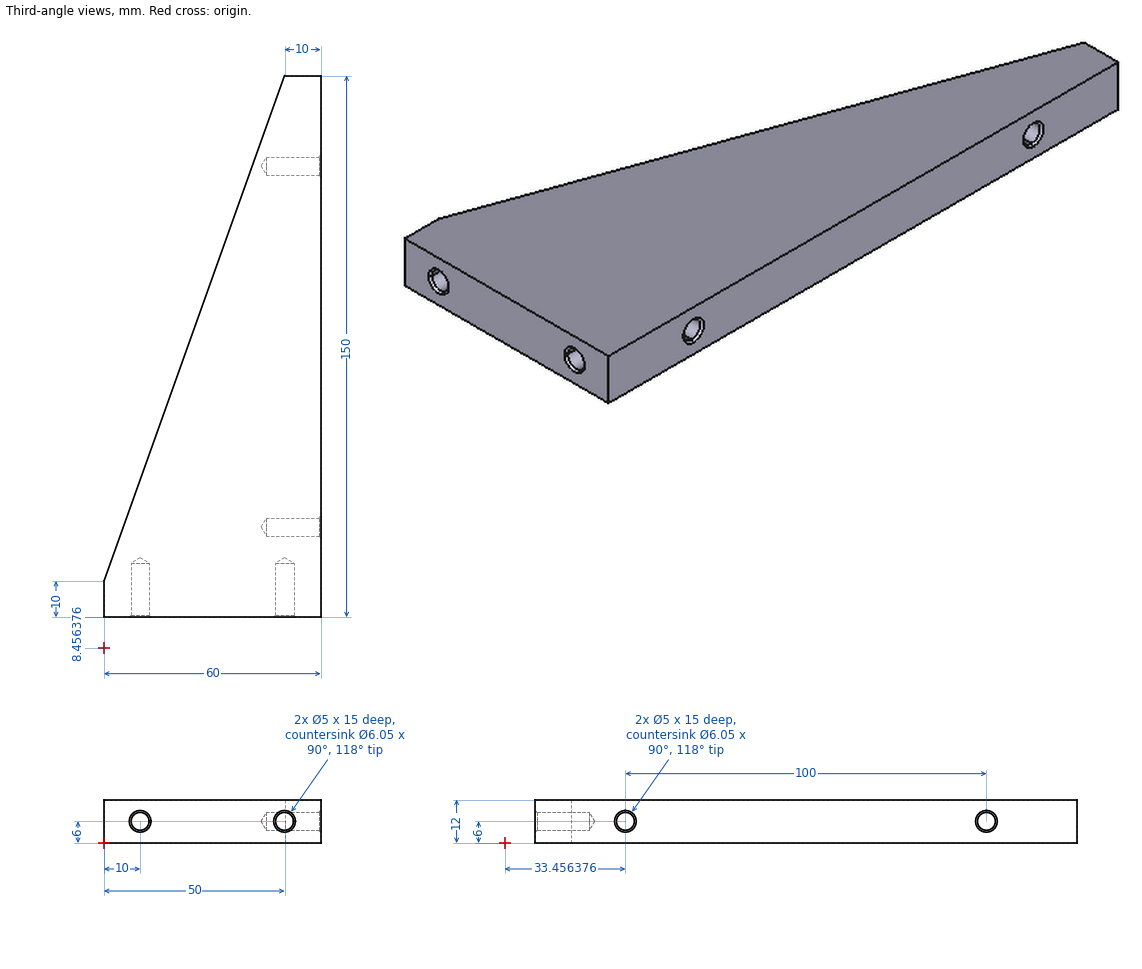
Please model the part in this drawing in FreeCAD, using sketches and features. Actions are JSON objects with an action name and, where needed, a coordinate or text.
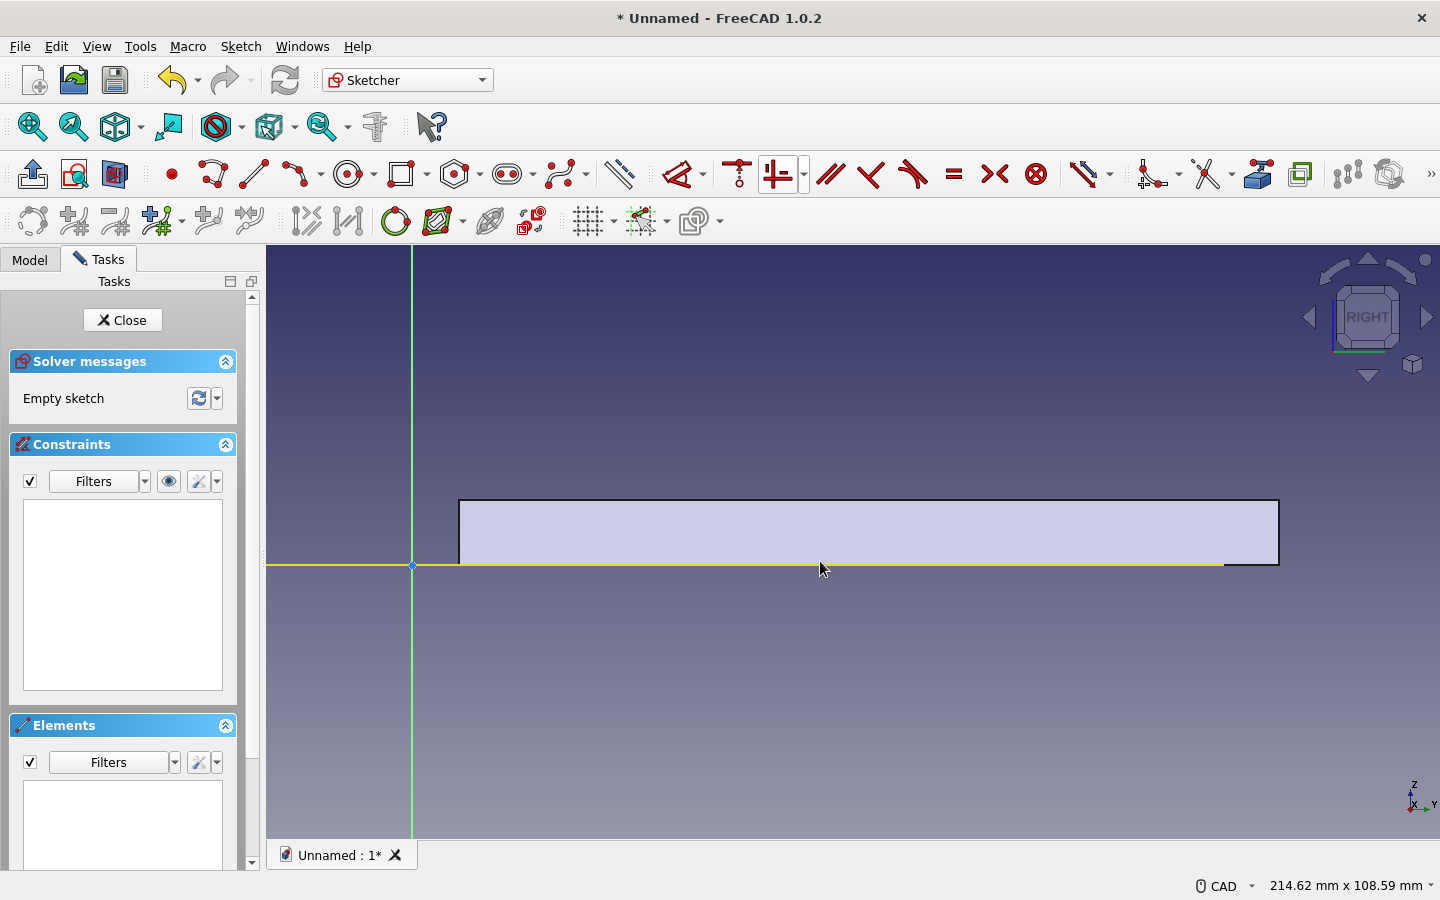
{"action": "left_click", "coordinate": [348, 174]}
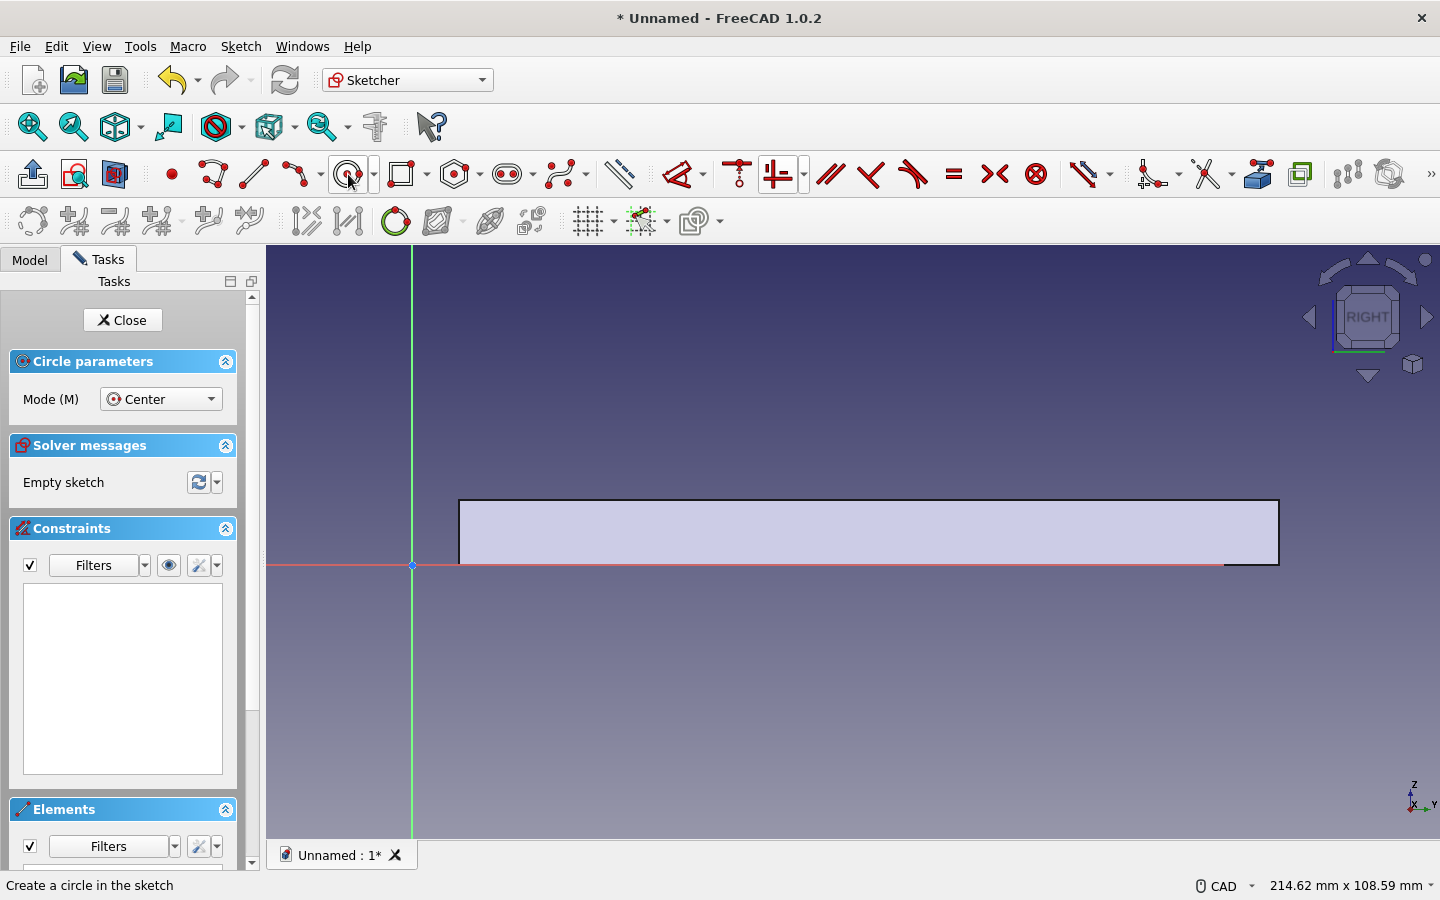
{"action": "scroll", "coordinate": [595, 532], "scroll_direction": "up", "scroll_amount": 3}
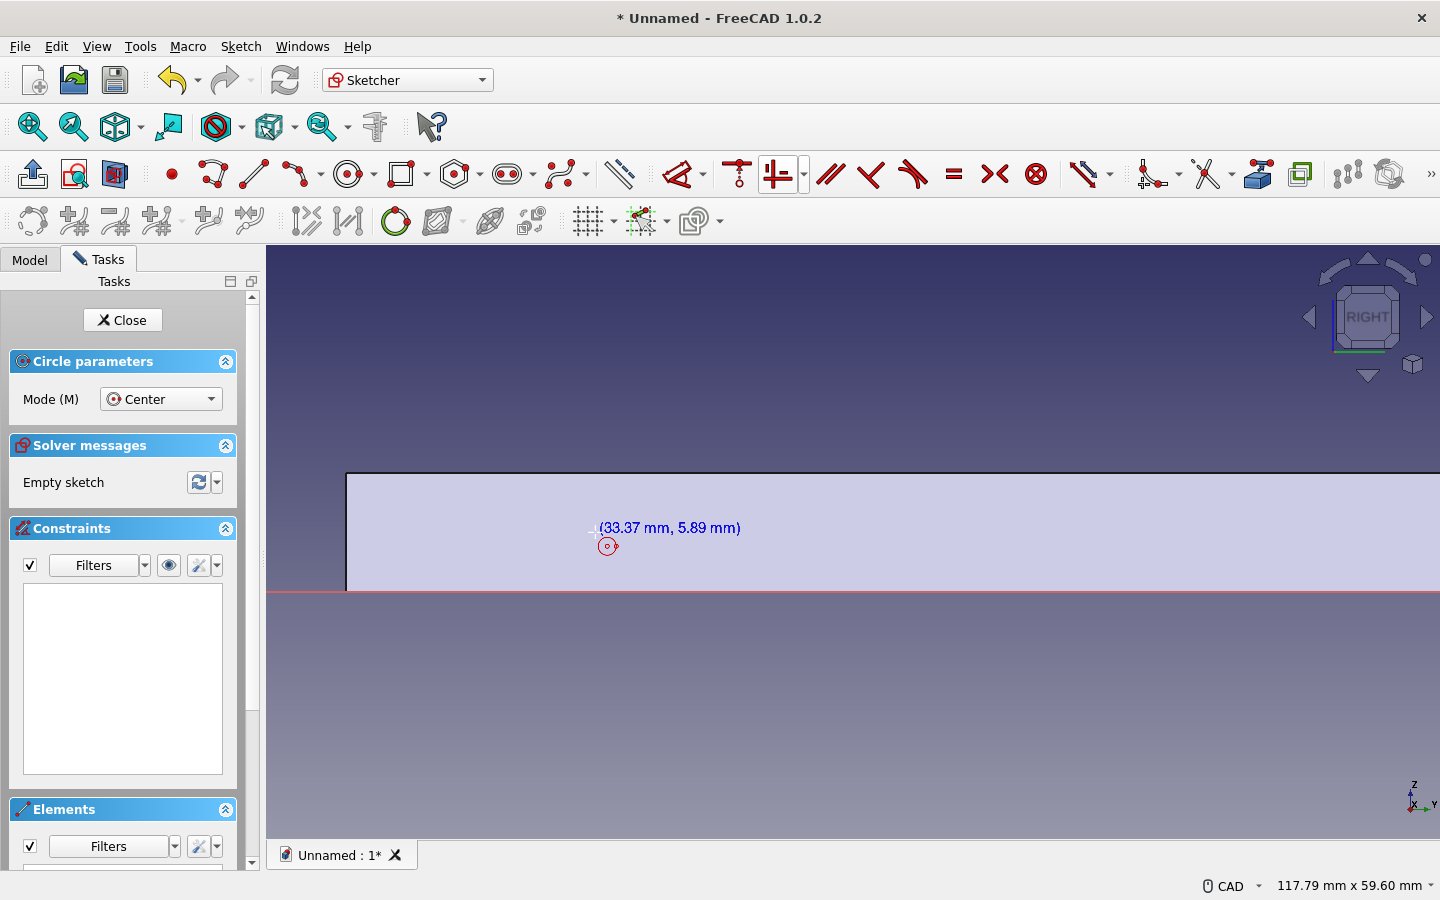
{"action": "left_click", "coordinate": [596, 532]}
{"action": "mouse_move", "coordinate": [613, 515]}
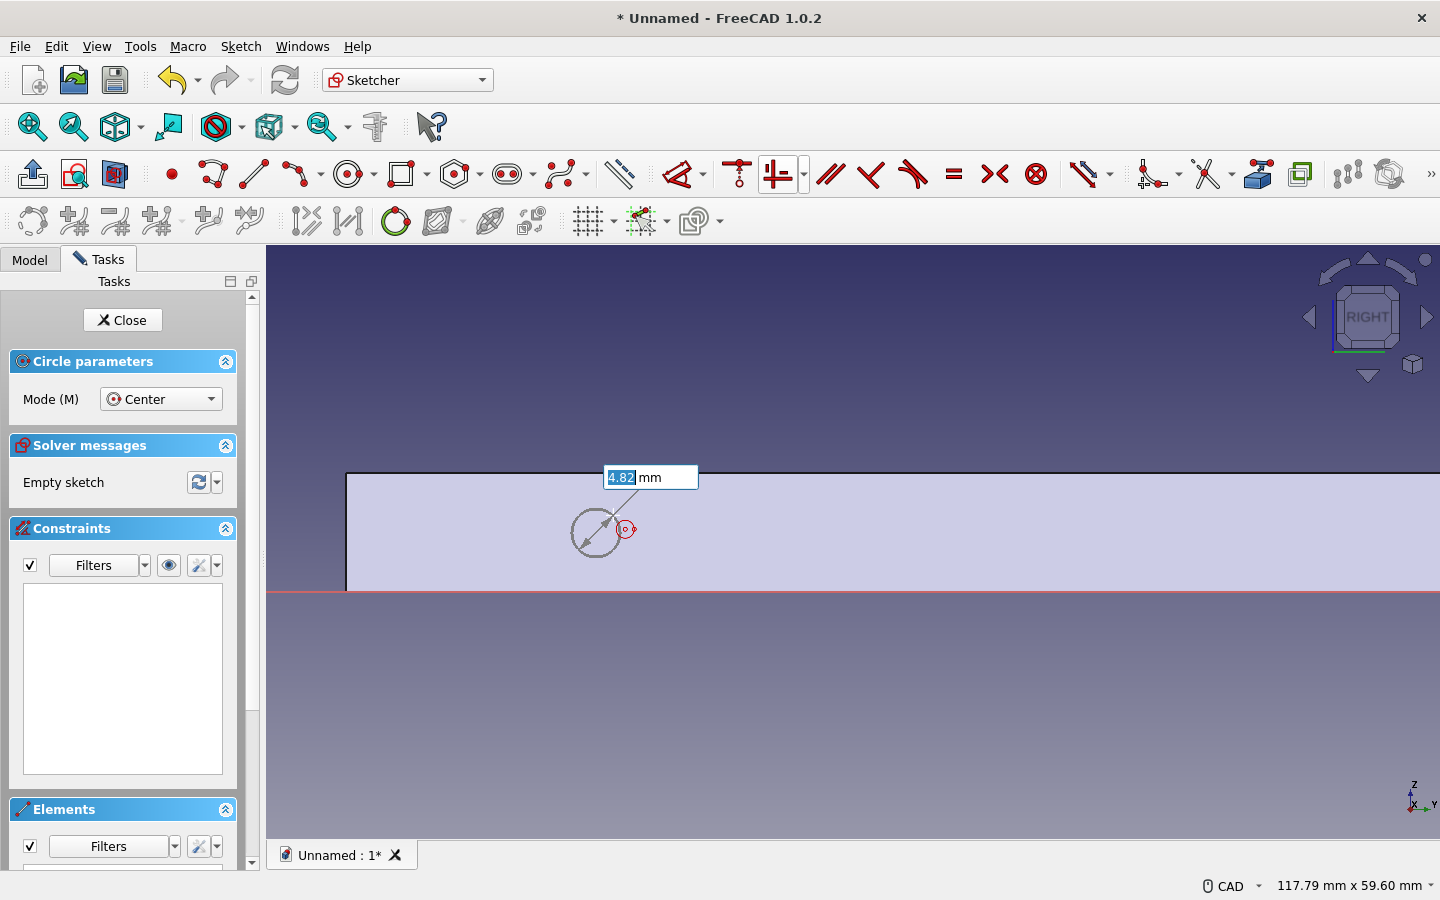
{"action": "type", "text": "5"}
{"action": "key", "text": "Return"}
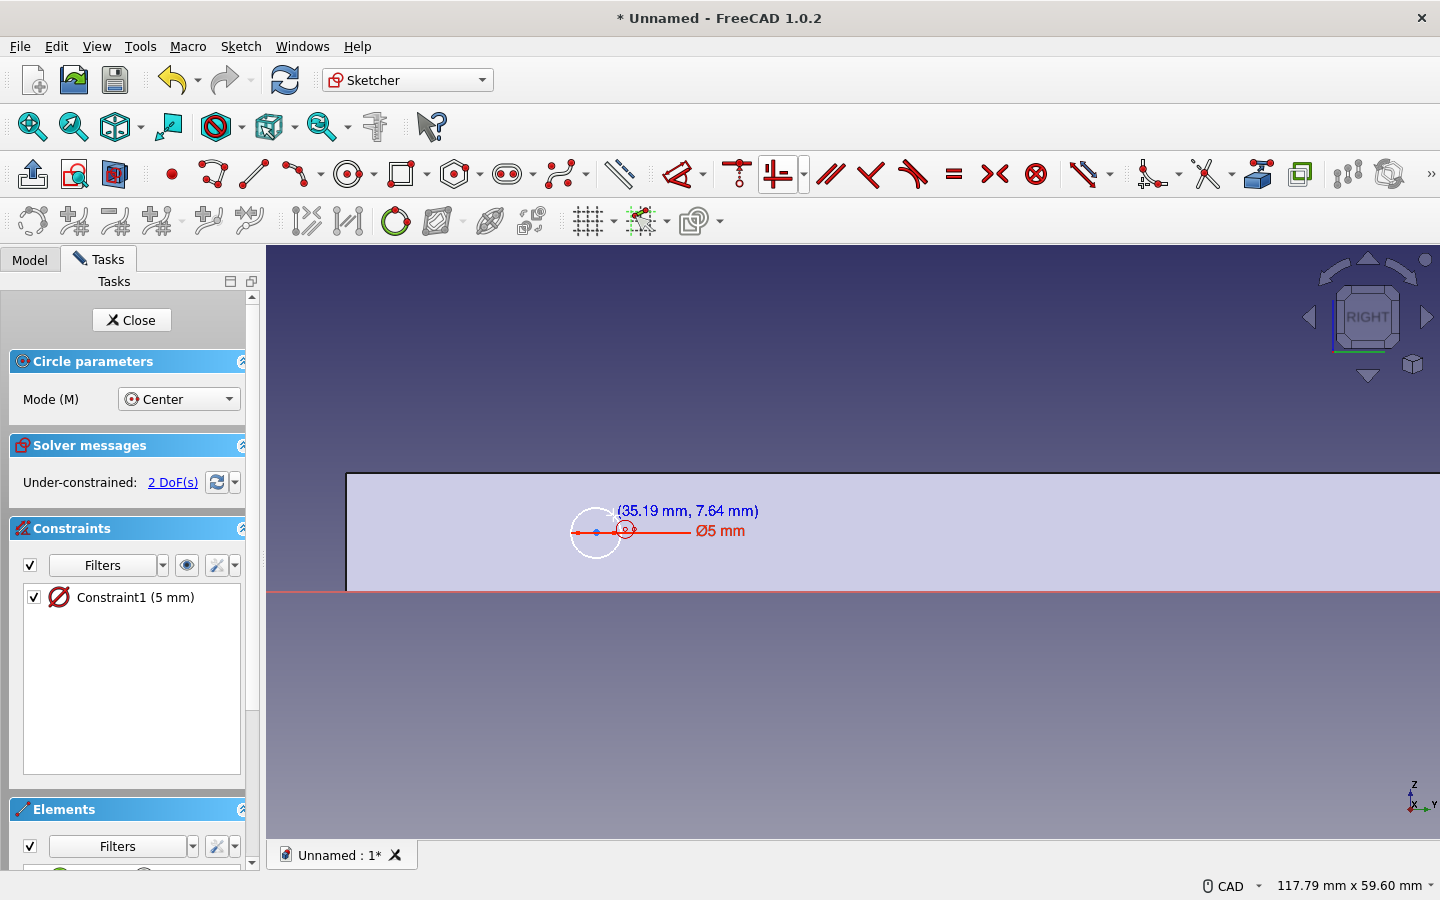
{"action": "scroll", "coordinate": [596, 533], "scroll_direction": "down", "scroll_amount": 3}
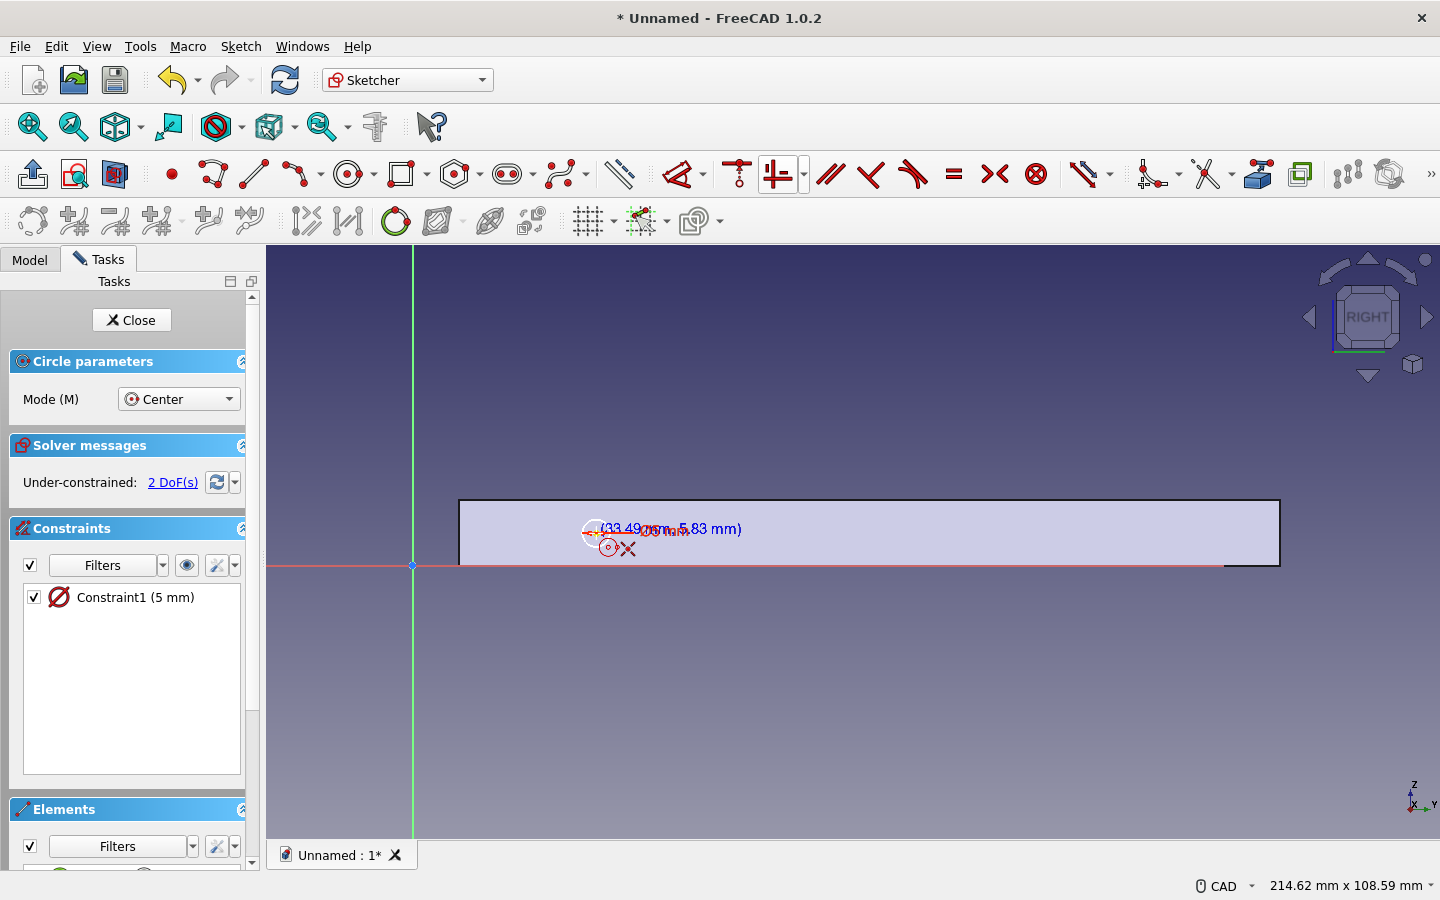
{"action": "scroll", "coordinate": [1143, 533], "scroll_direction": "up", "scroll_amount": 3}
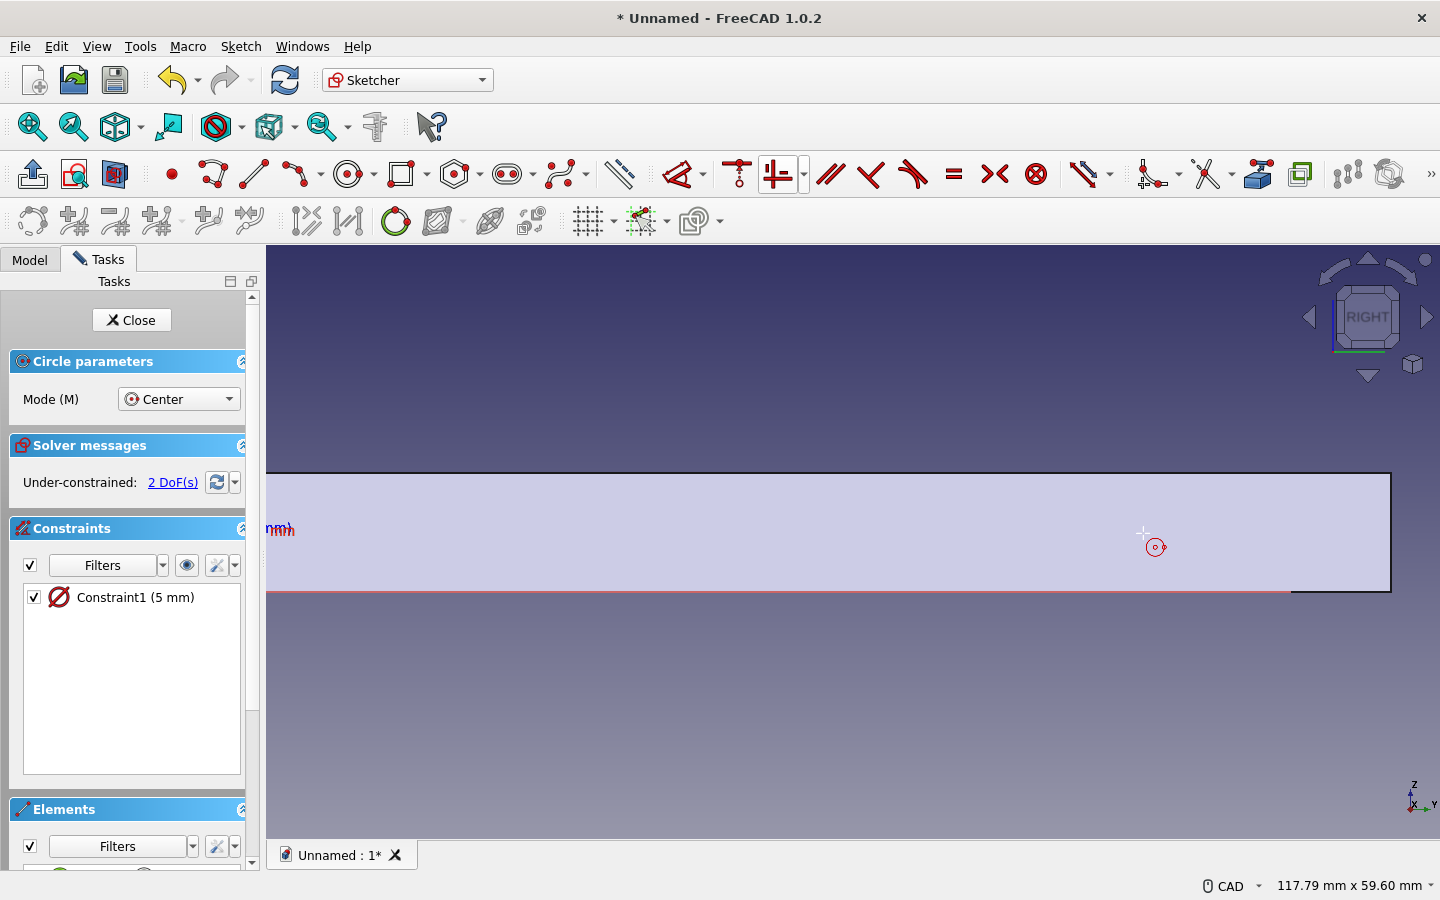
{"action": "left_click", "coordinate": [1142, 532]}
{"action": "mouse_move", "coordinate": [1160, 515]}